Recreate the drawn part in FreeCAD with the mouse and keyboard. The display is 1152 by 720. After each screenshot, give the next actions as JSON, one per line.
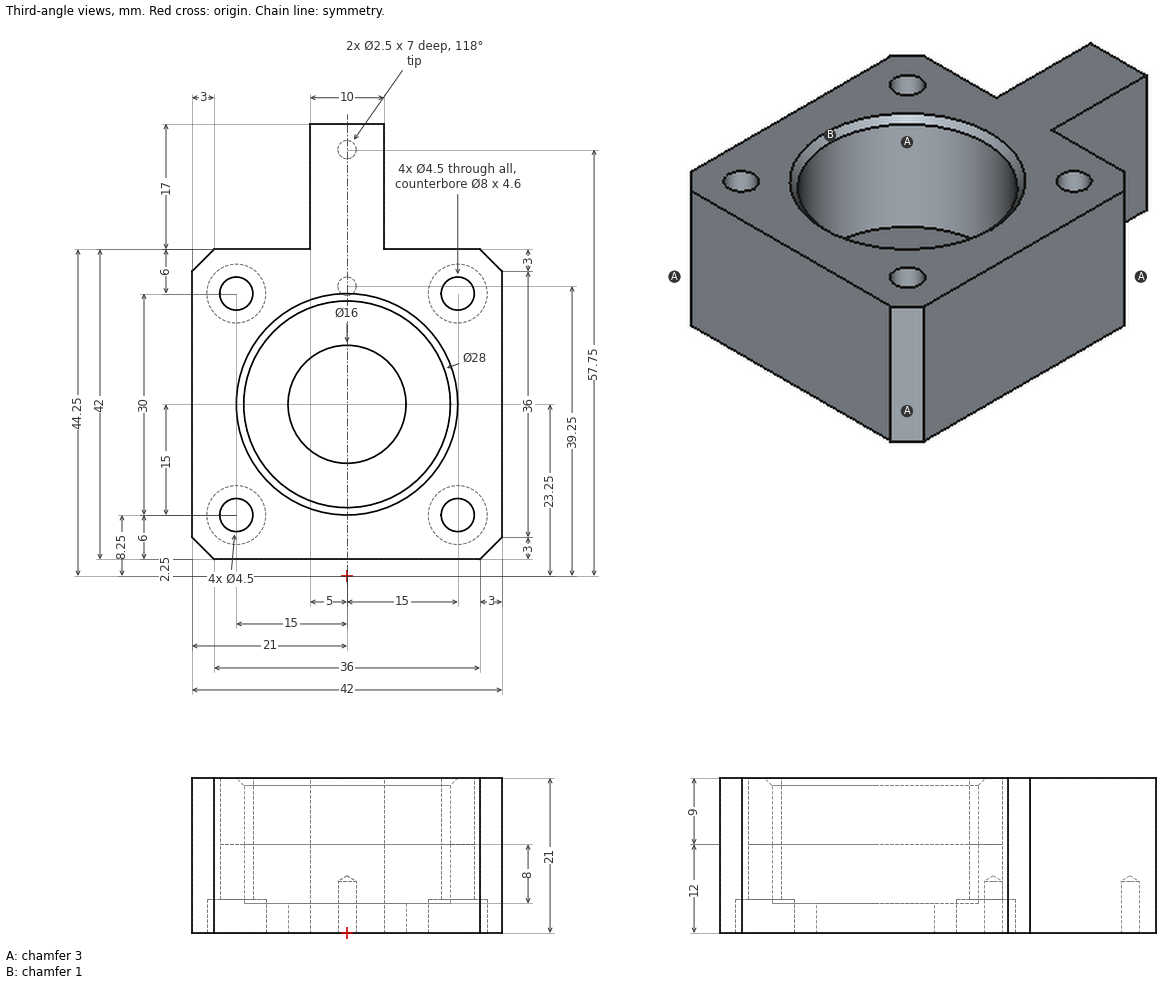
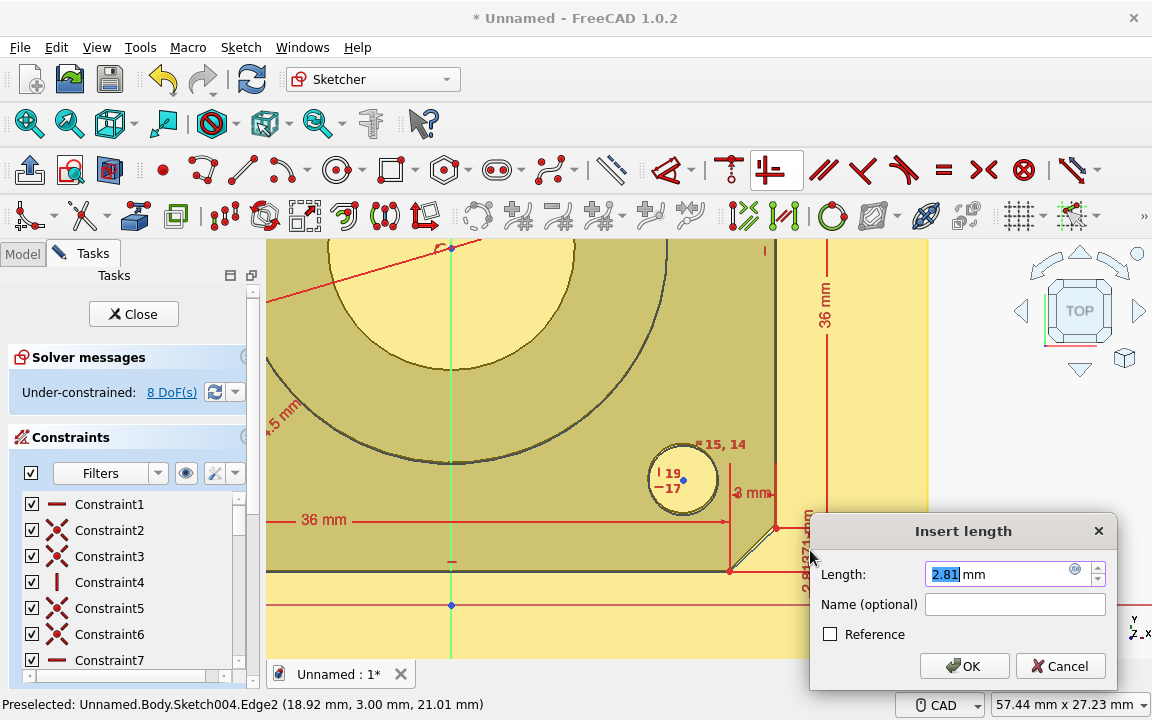
{"action": "type", "text": "3"}
{"action": "key", "text": "Return"}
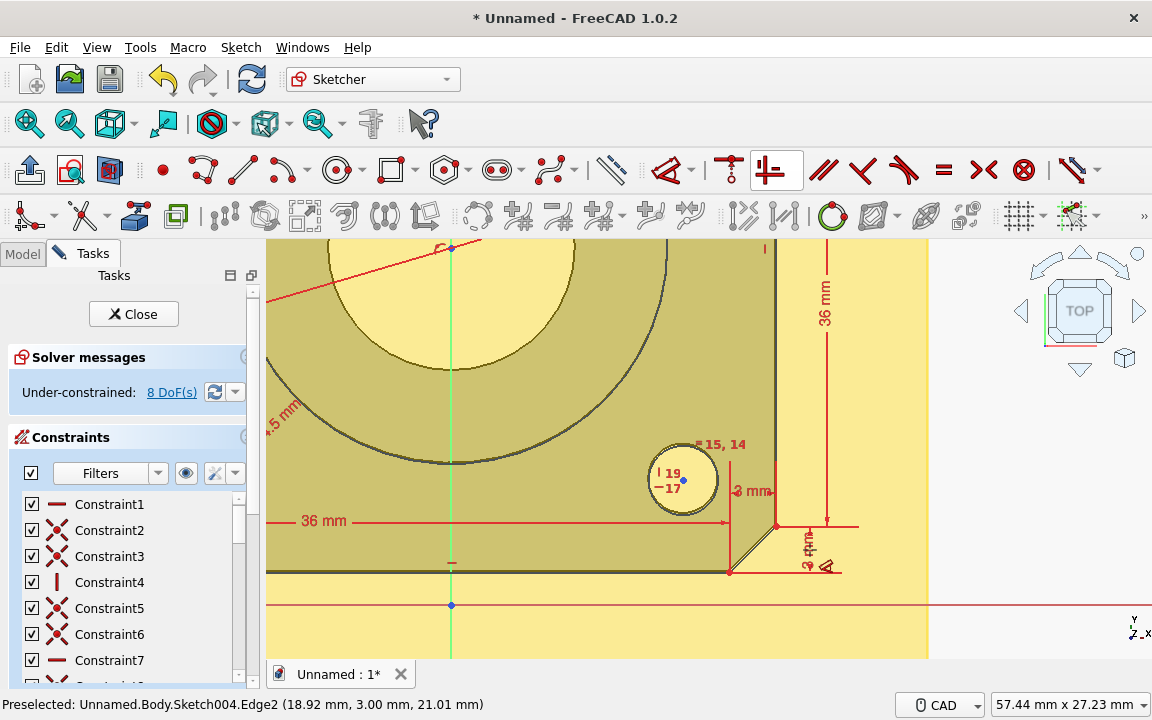
{"action": "scroll", "coordinate": [751, 557], "scroll_direction": "down", "scroll_amount": 5}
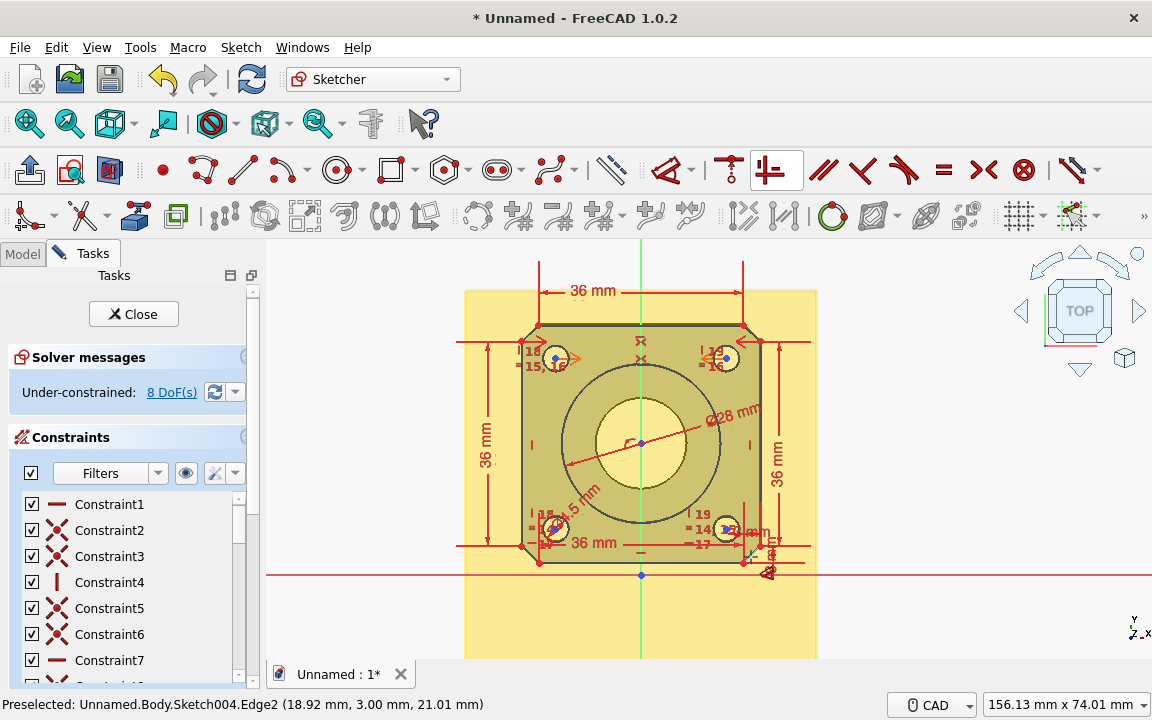
{"action": "scroll", "coordinate": [755, 337], "scroll_direction": "up", "scroll_amount": 5}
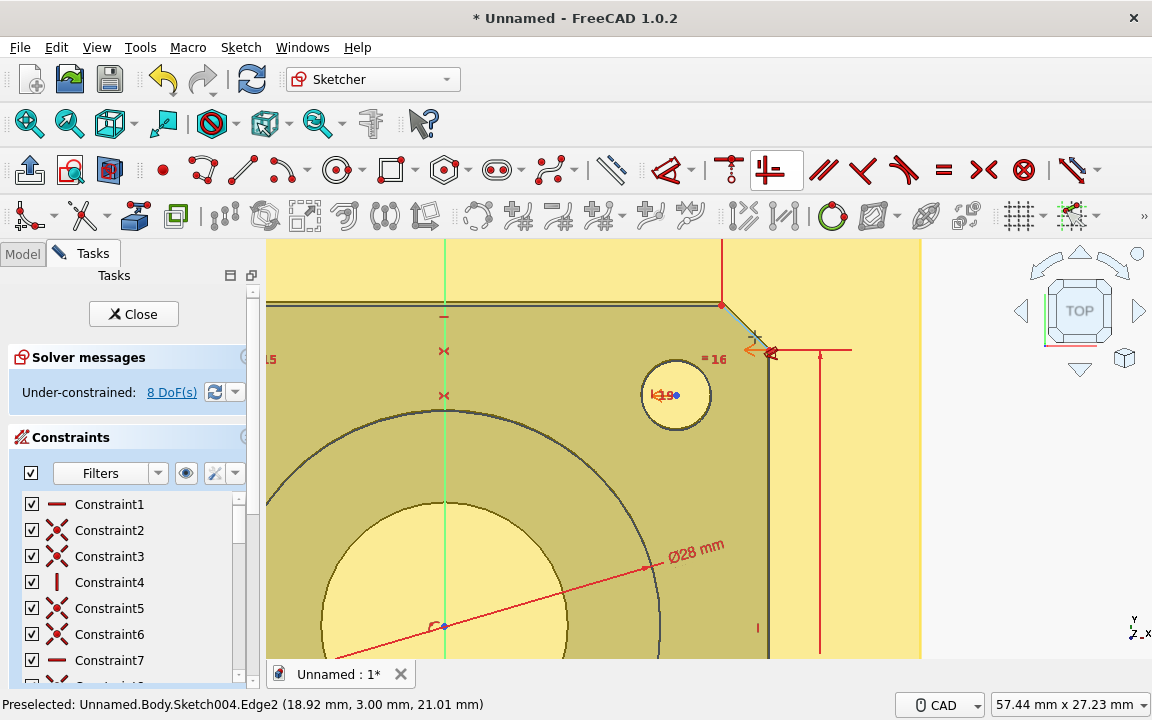
{"action": "left_click", "coordinate": [755, 337]}
{"action": "left_click", "coordinate": [745, 272]}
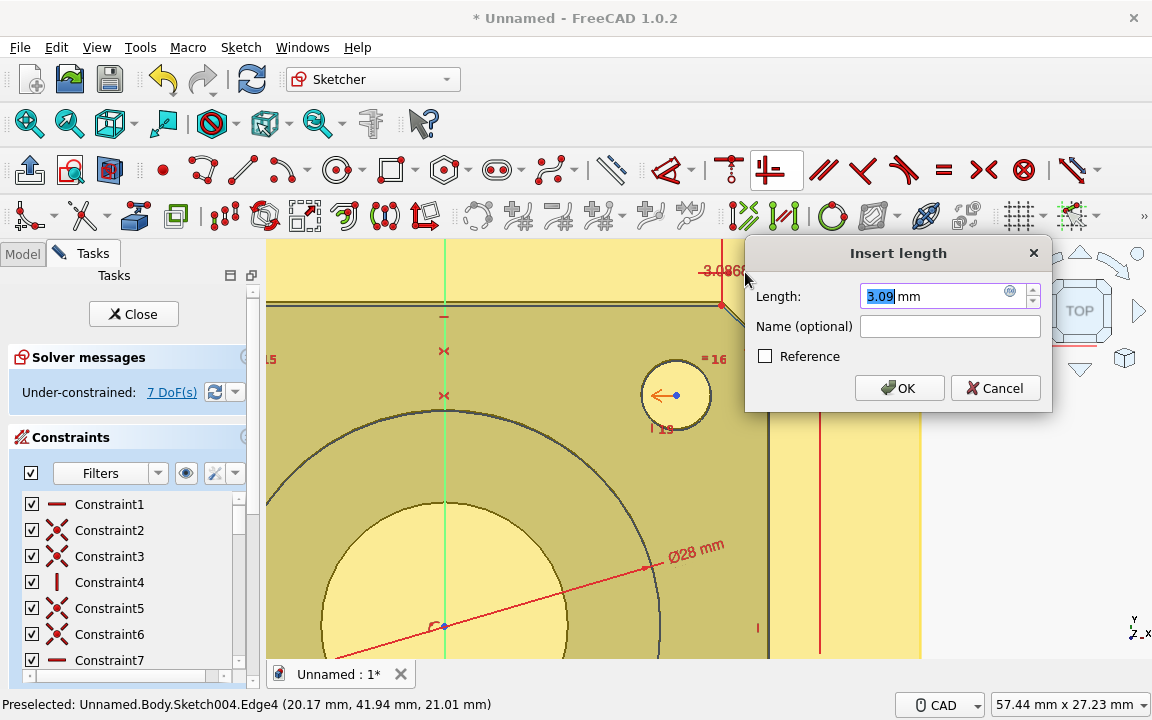
{"action": "type", "text": "3"}
{"action": "key", "text": "Return"}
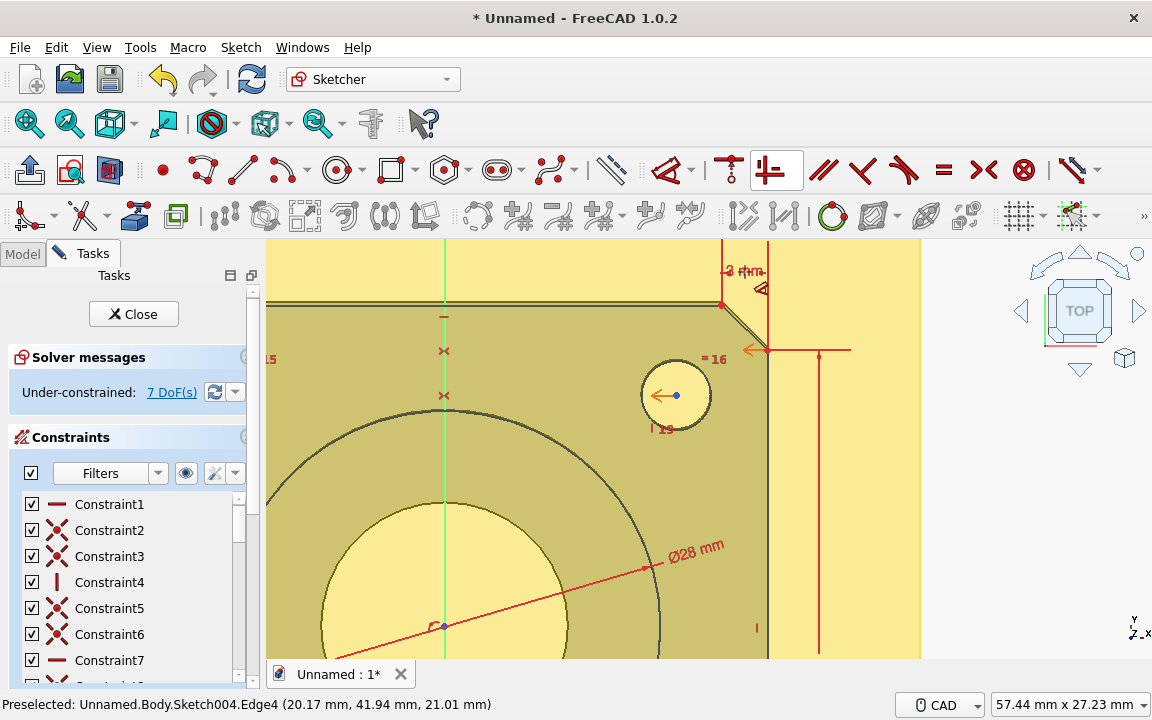
{"action": "left_click", "coordinate": [754, 337]}
{"action": "left_click", "coordinate": [802, 328]}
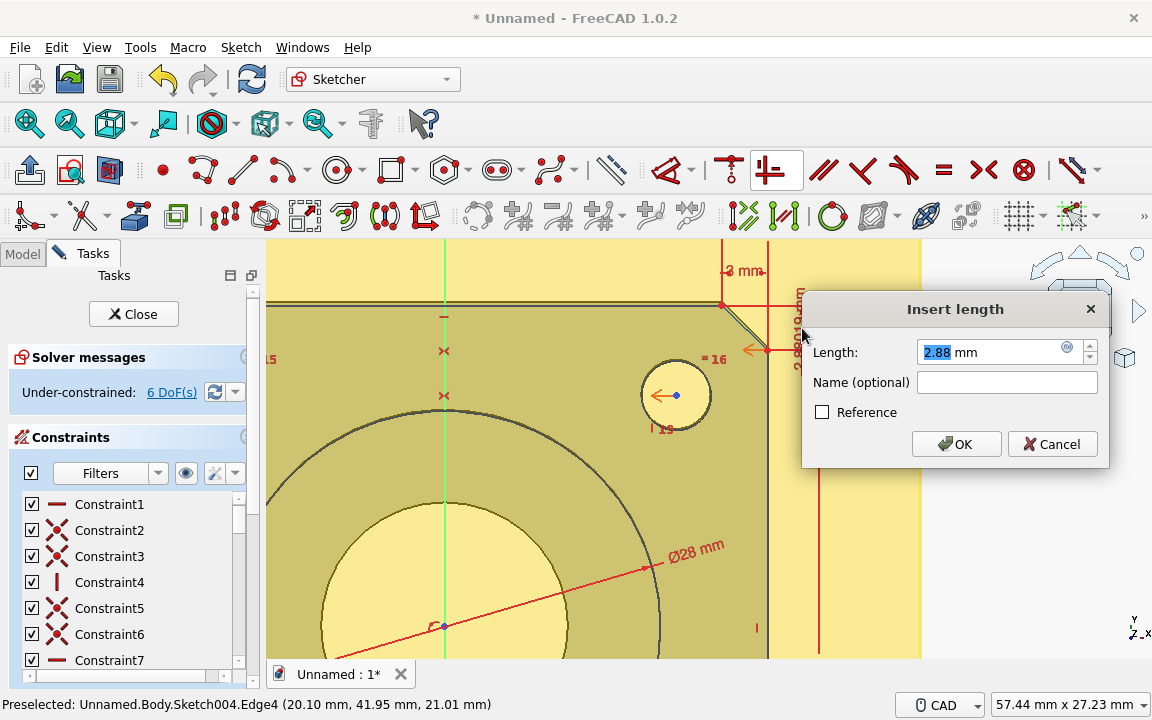
{"action": "type", "text": "3"}
{"action": "key", "text": "Return"}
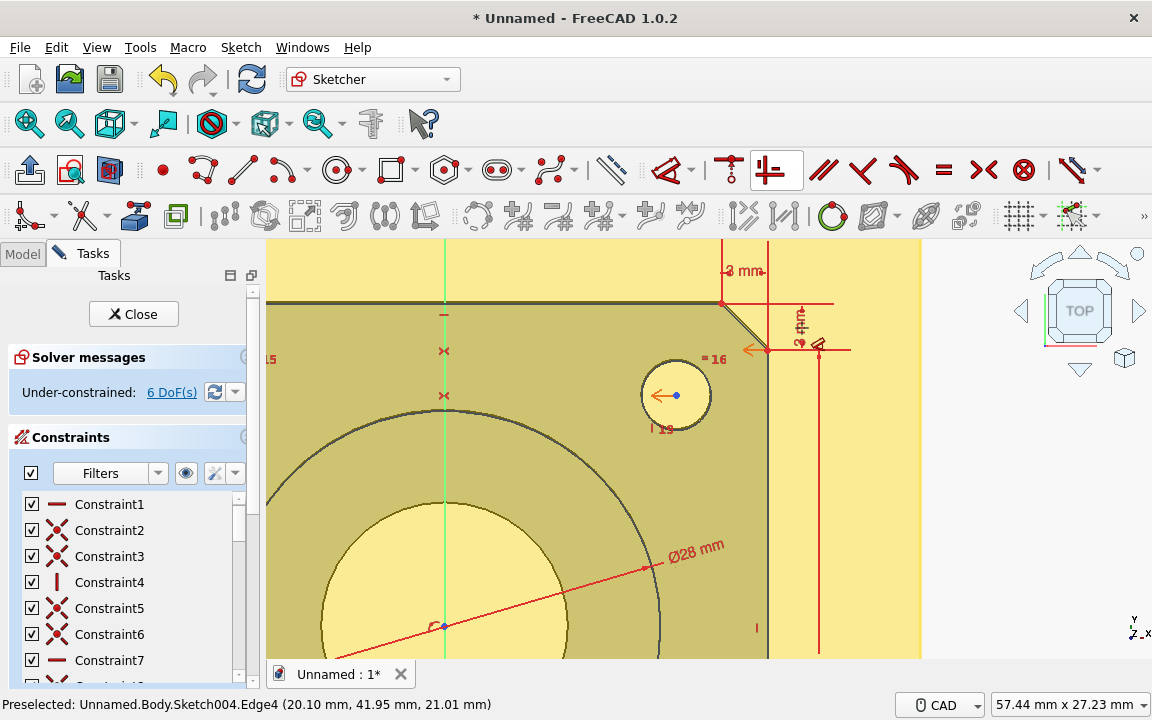
{"action": "scroll", "coordinate": [755, 336], "scroll_direction": "down", "scroll_amount": 5}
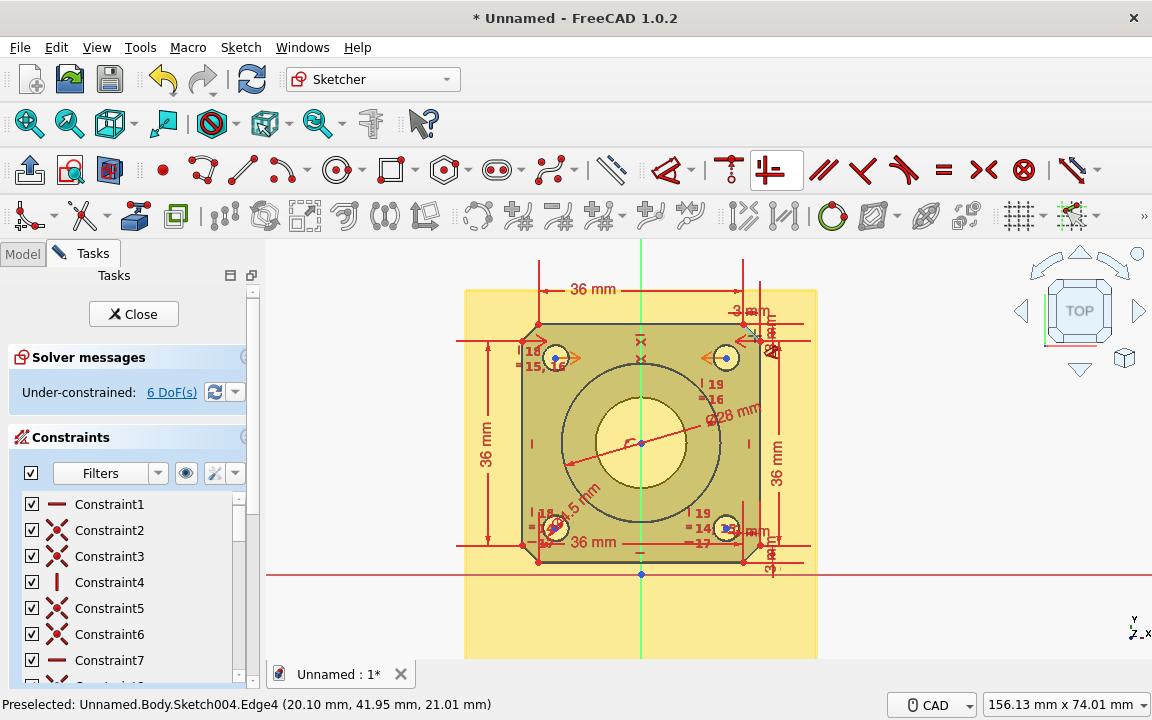
{"action": "scroll", "coordinate": [534, 329], "scroll_direction": "up", "scroll_amount": 5}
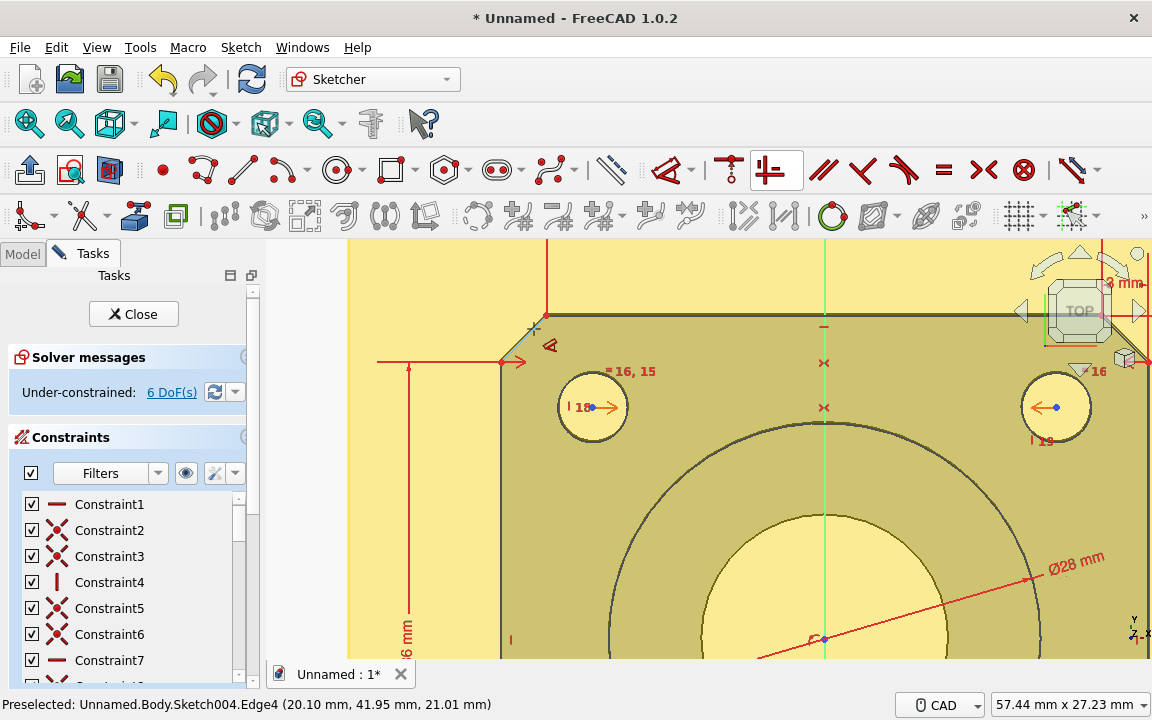
{"action": "left_click", "coordinate": [533, 330]}
{"action": "left_click", "coordinate": [524, 282]}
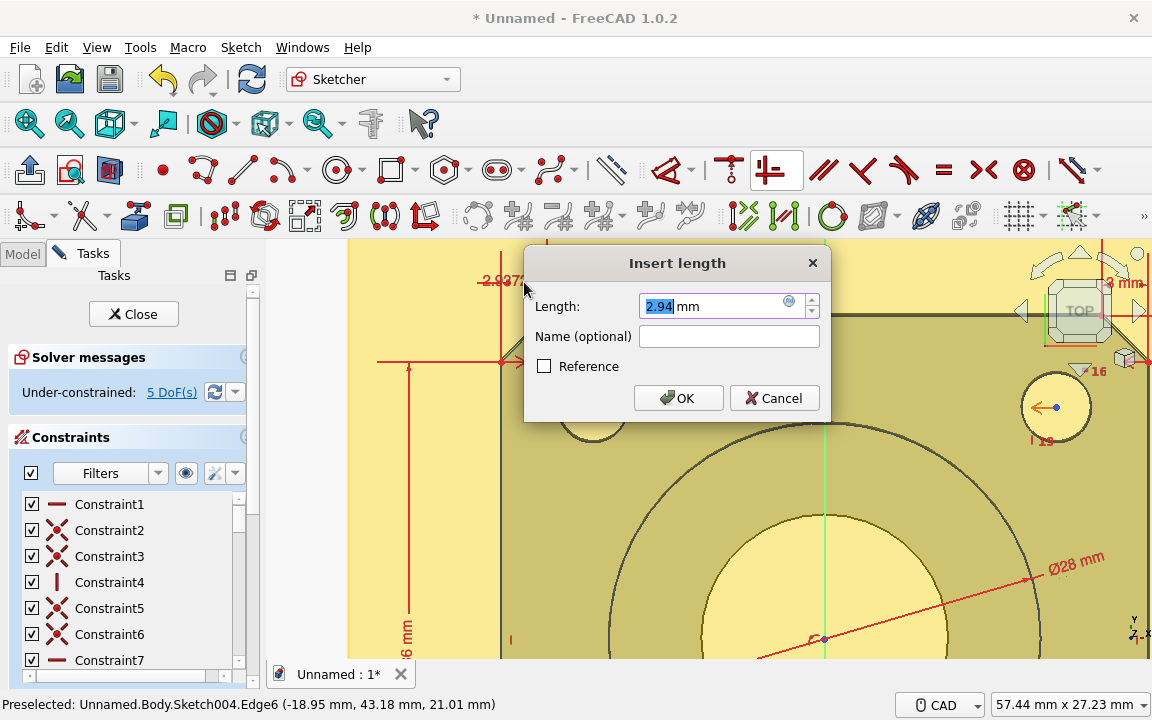
{"action": "type", "text": "3"}
{"action": "key", "text": "Return"}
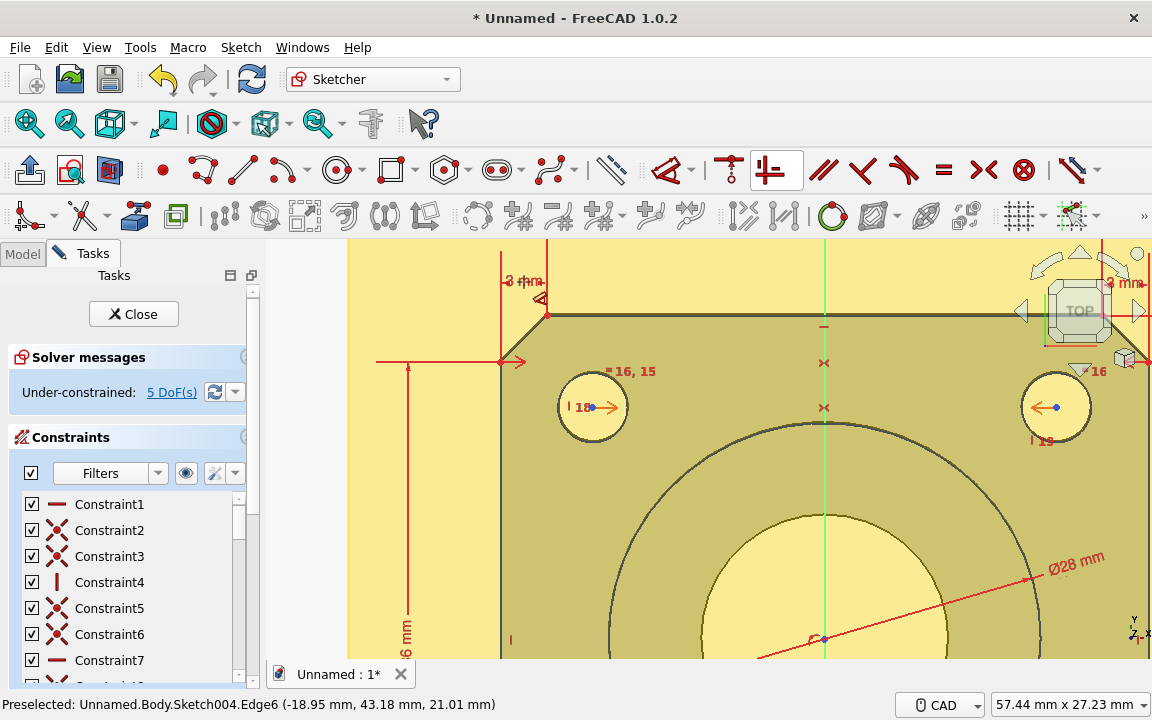
{"action": "scroll", "coordinate": [533, 329], "scroll_direction": "down", "scroll_amount": 5}